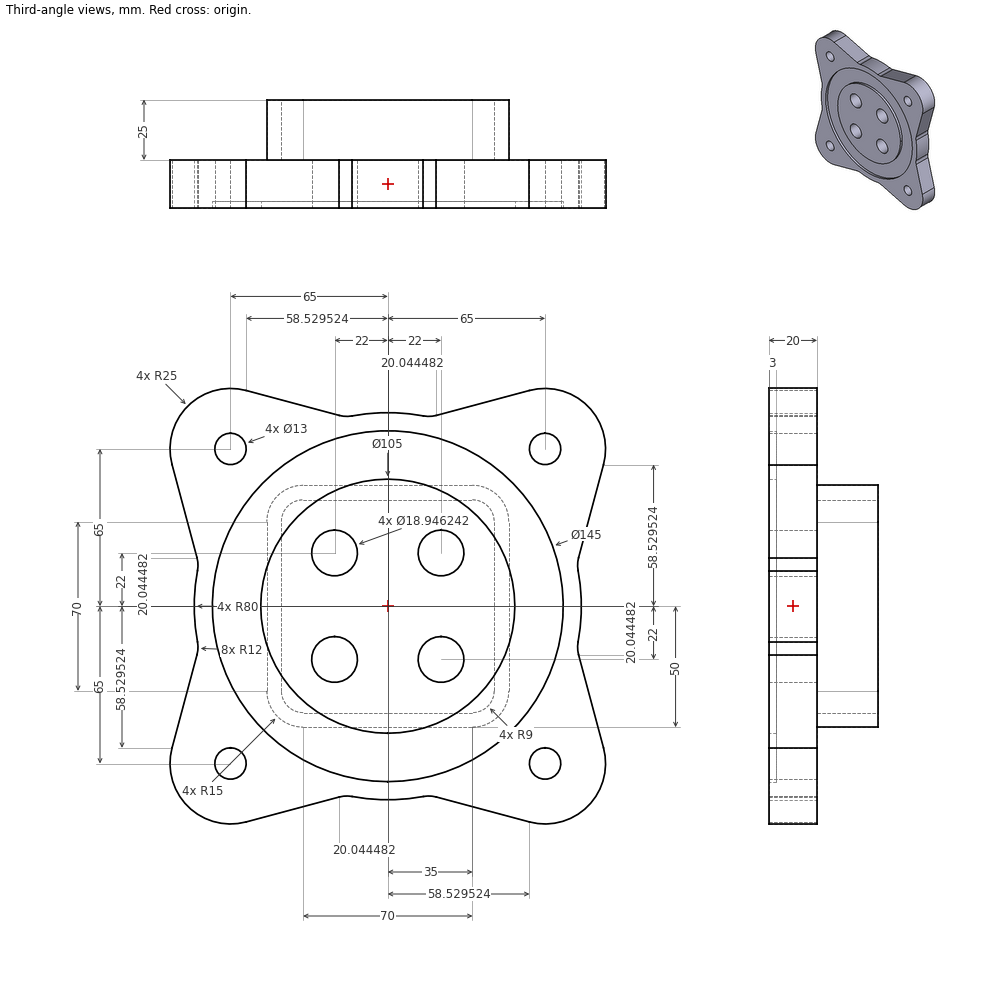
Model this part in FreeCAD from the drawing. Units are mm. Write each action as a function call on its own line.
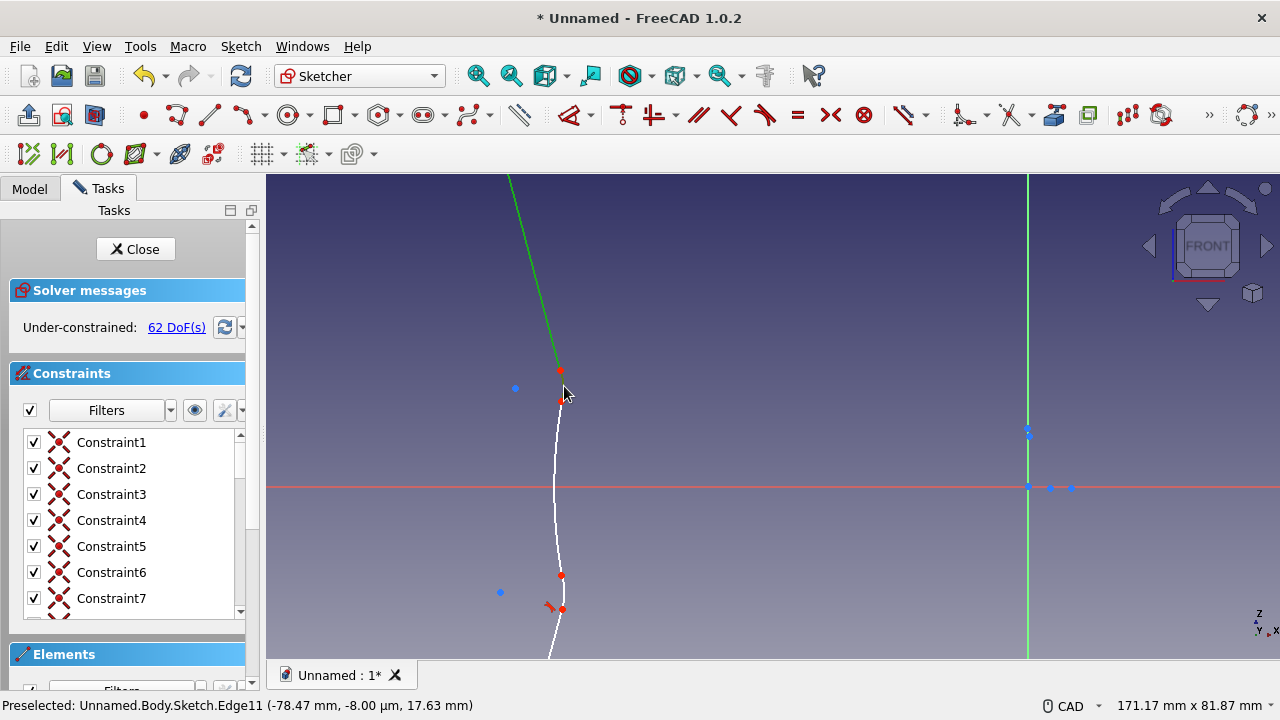
click(765, 116)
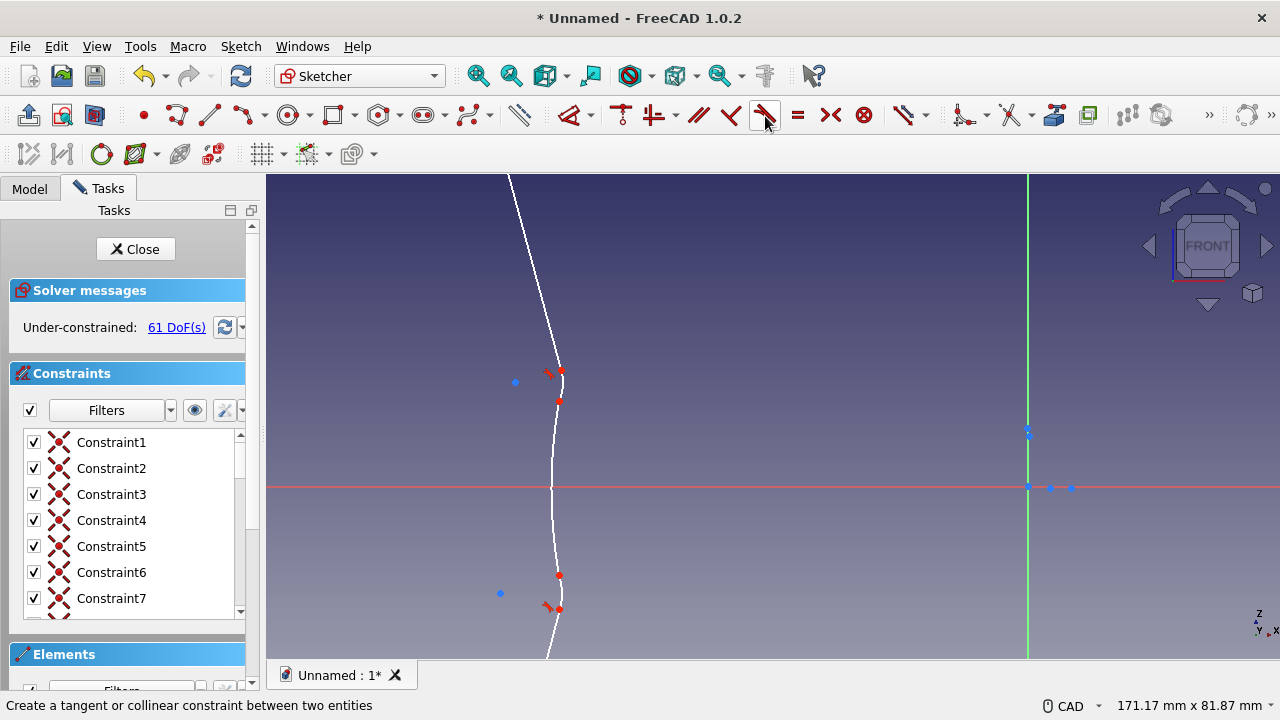
click(543, 303)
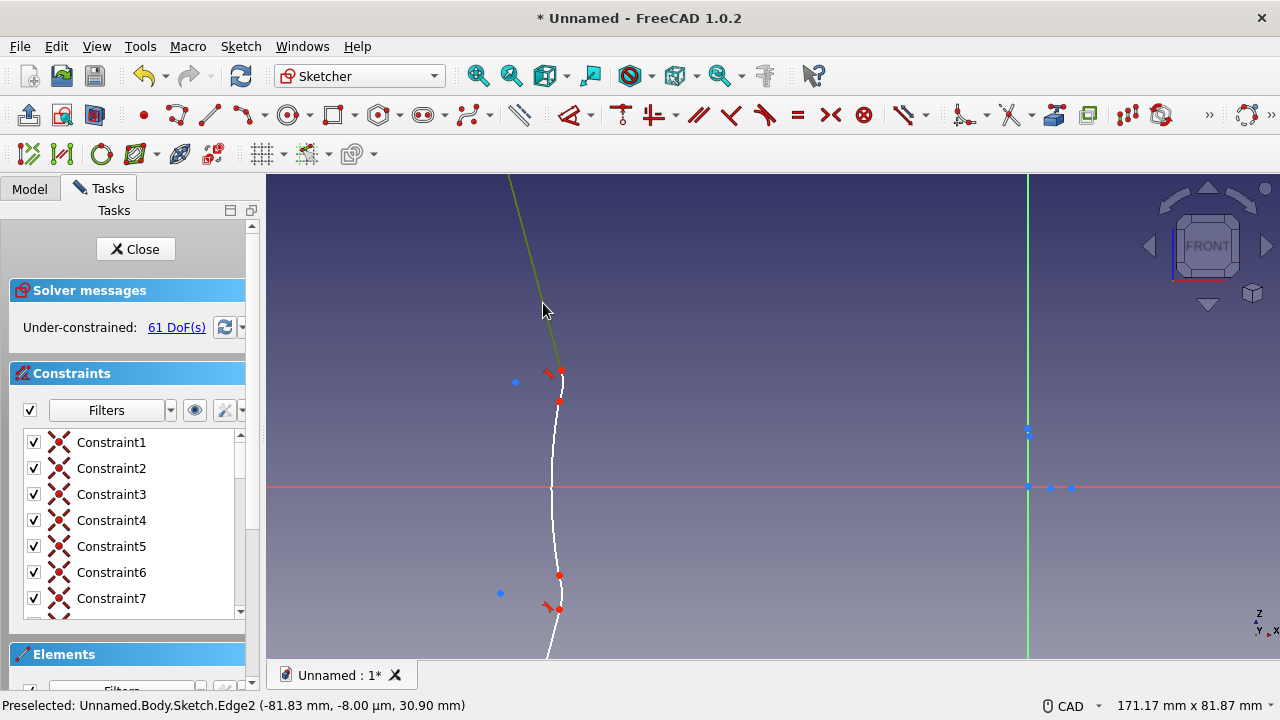
scroll(565, 386, down, 6)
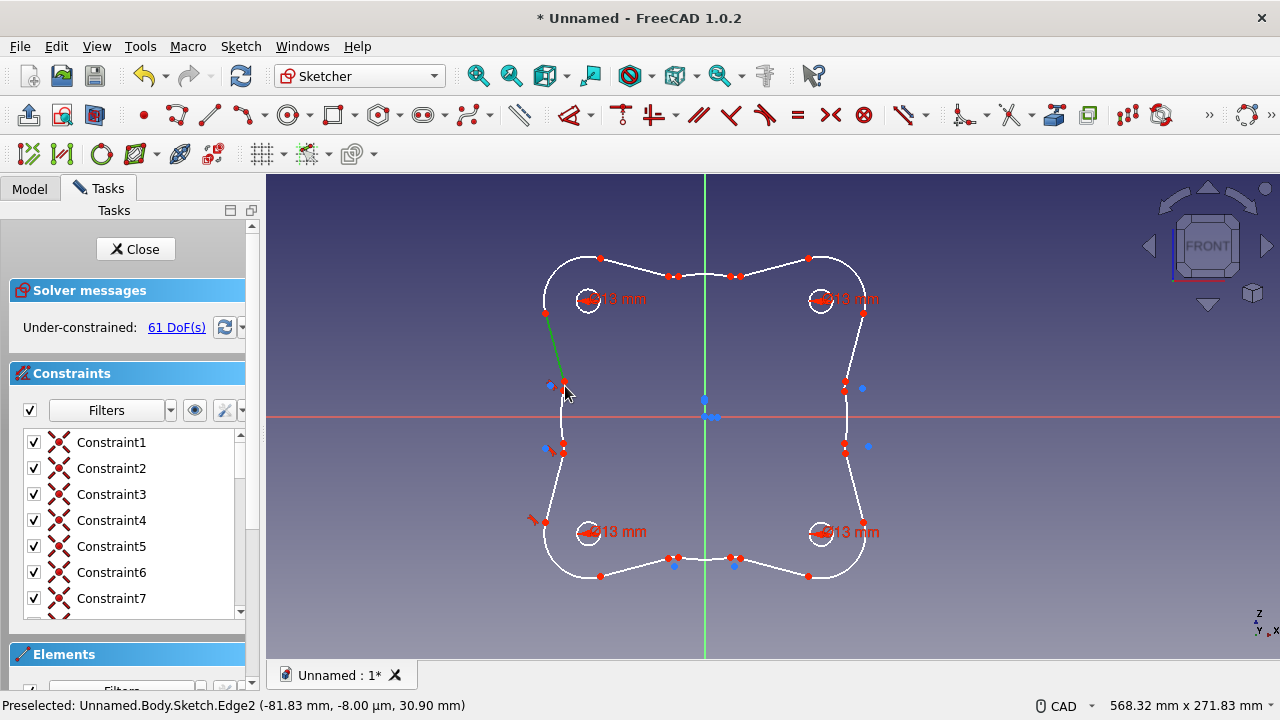
click(573, 260)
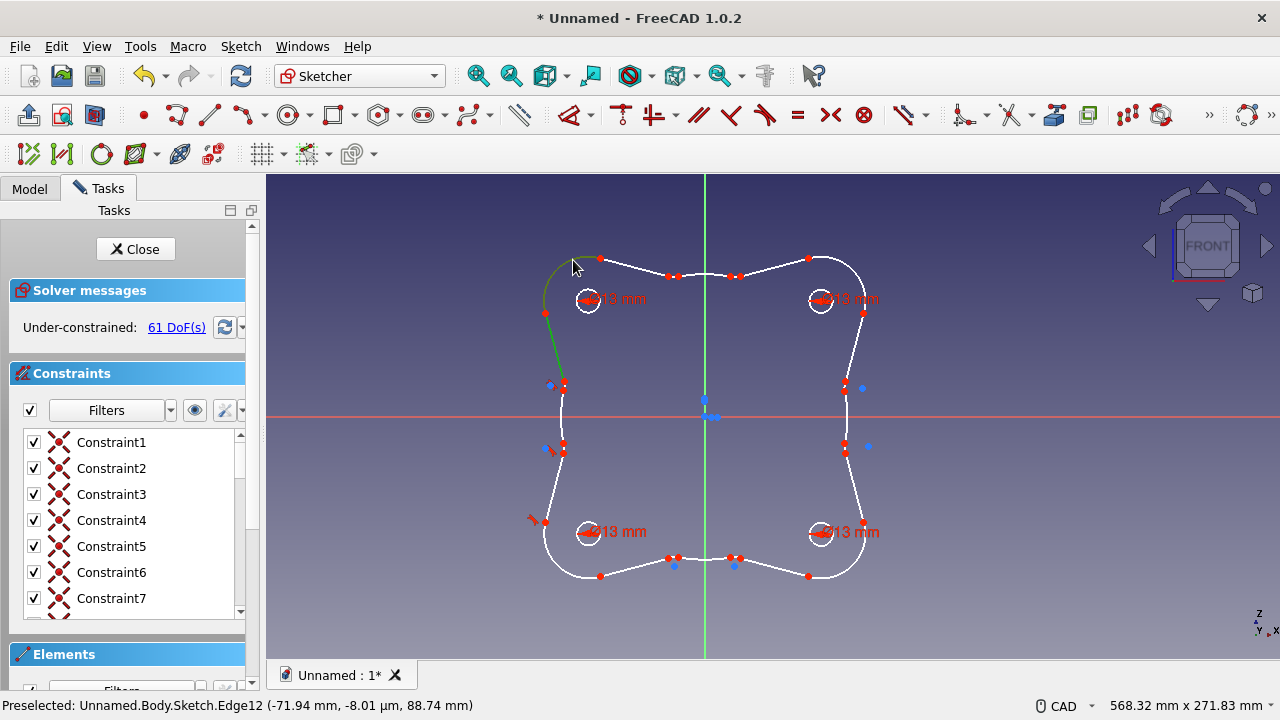
click(765, 116)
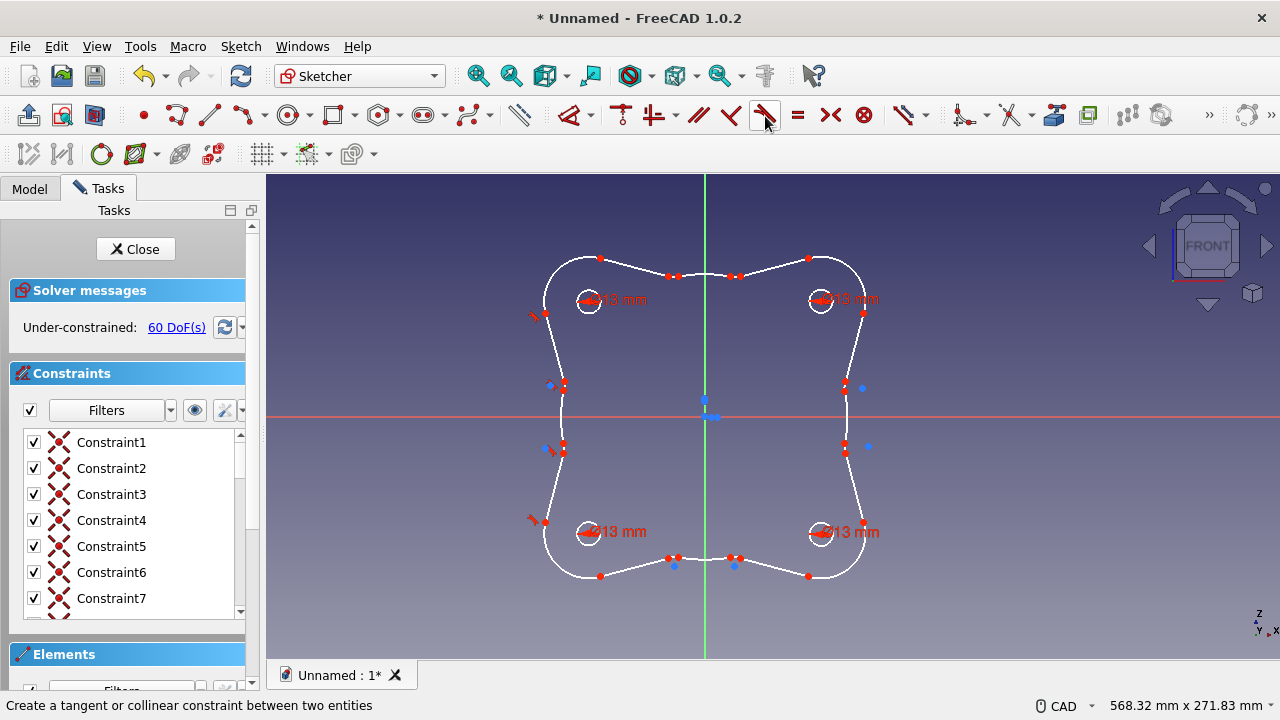
click(621, 264)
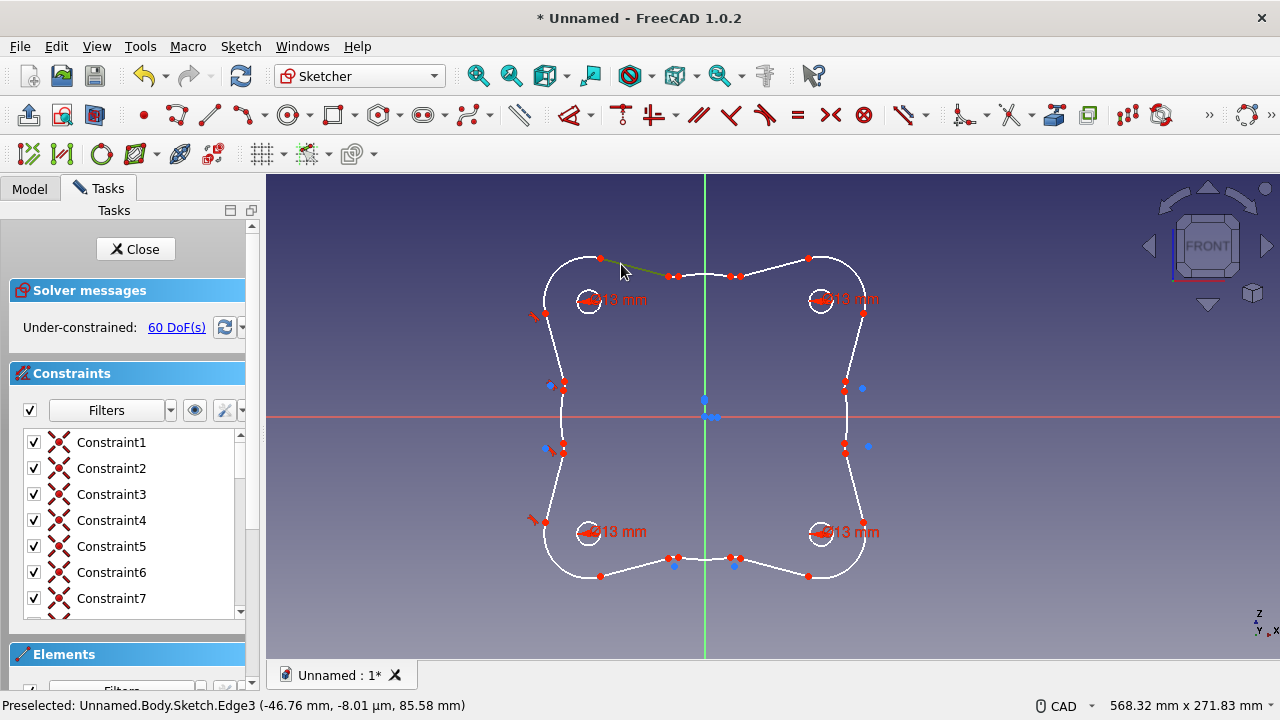
click(573, 260)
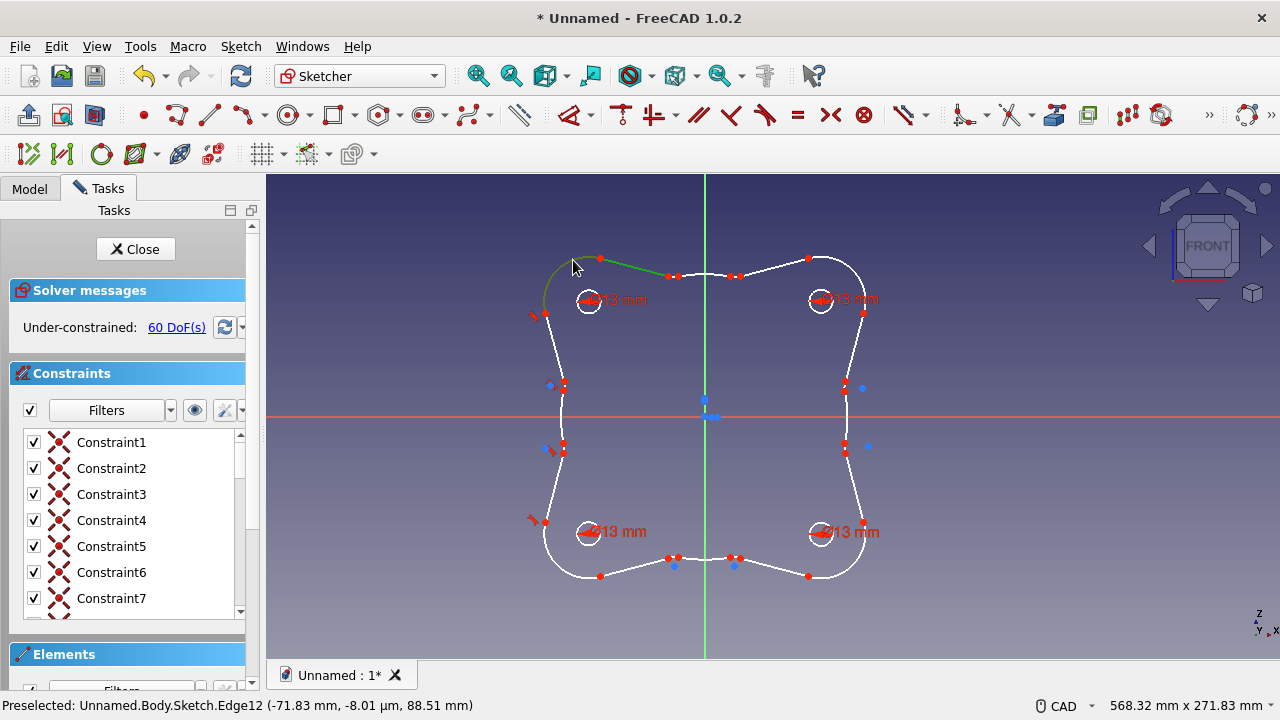
click(765, 116)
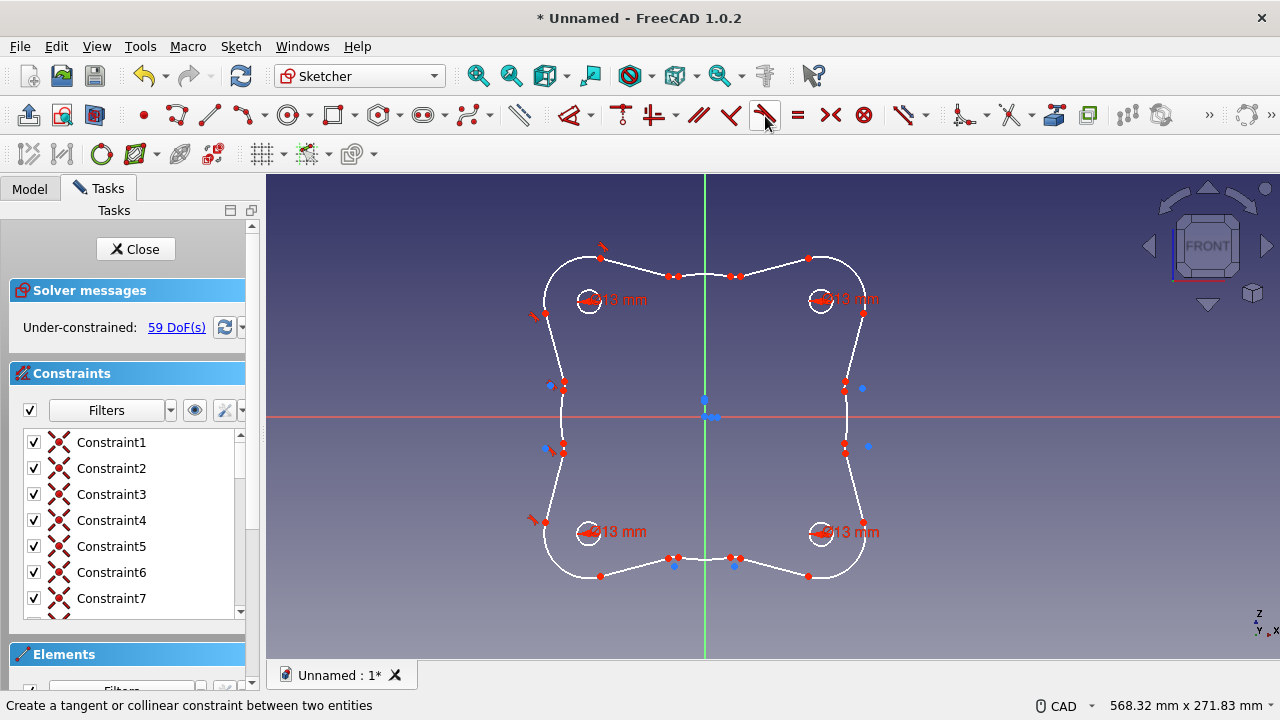
click(621, 264)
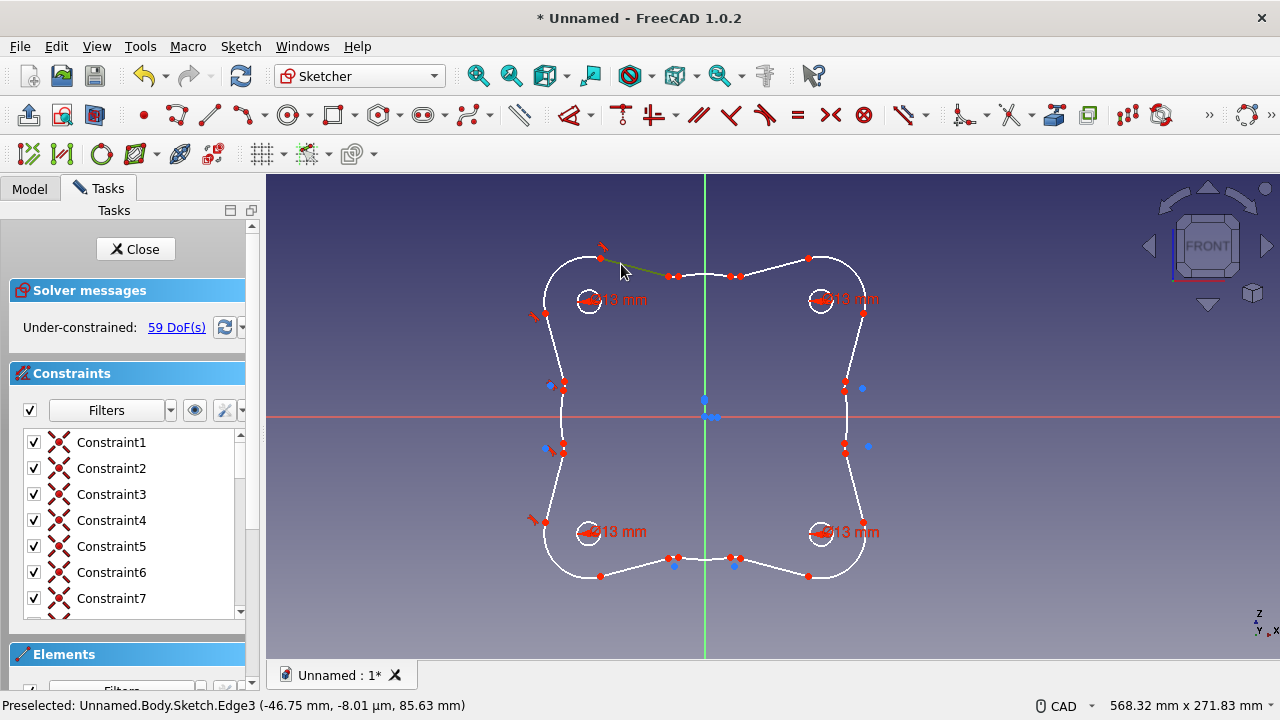
scroll(674, 277, up, 6)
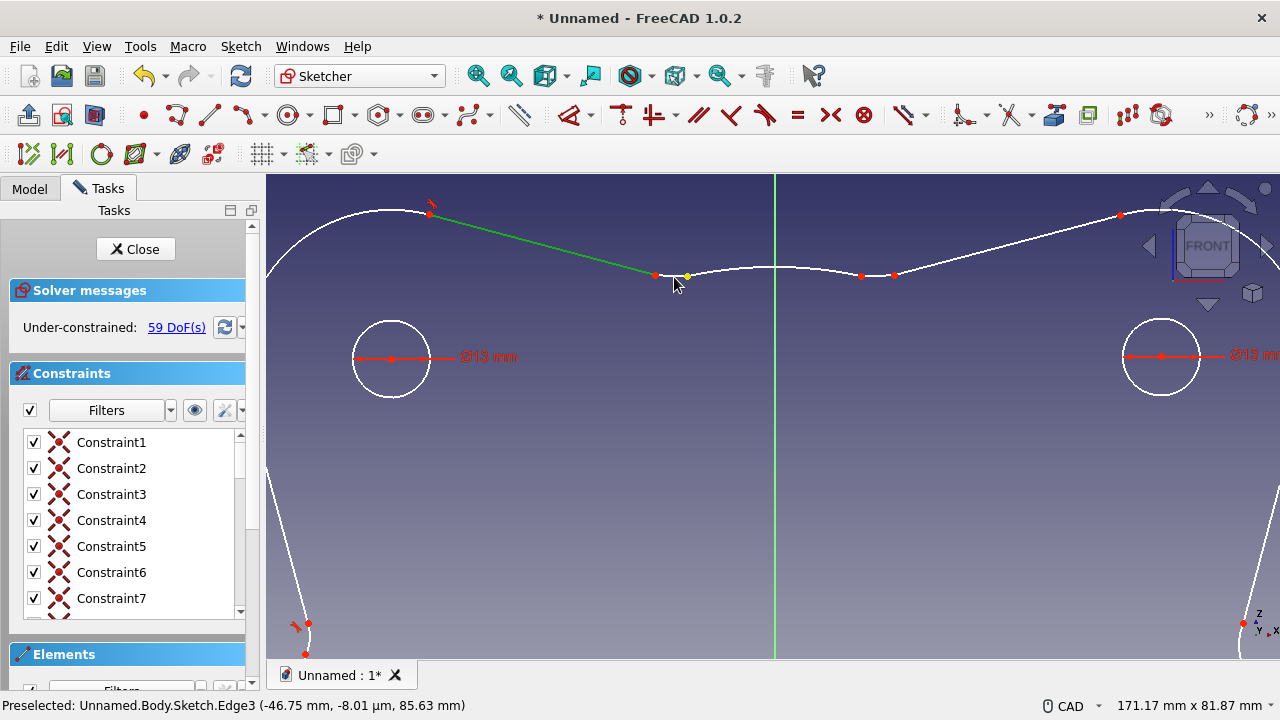
click(672, 276)